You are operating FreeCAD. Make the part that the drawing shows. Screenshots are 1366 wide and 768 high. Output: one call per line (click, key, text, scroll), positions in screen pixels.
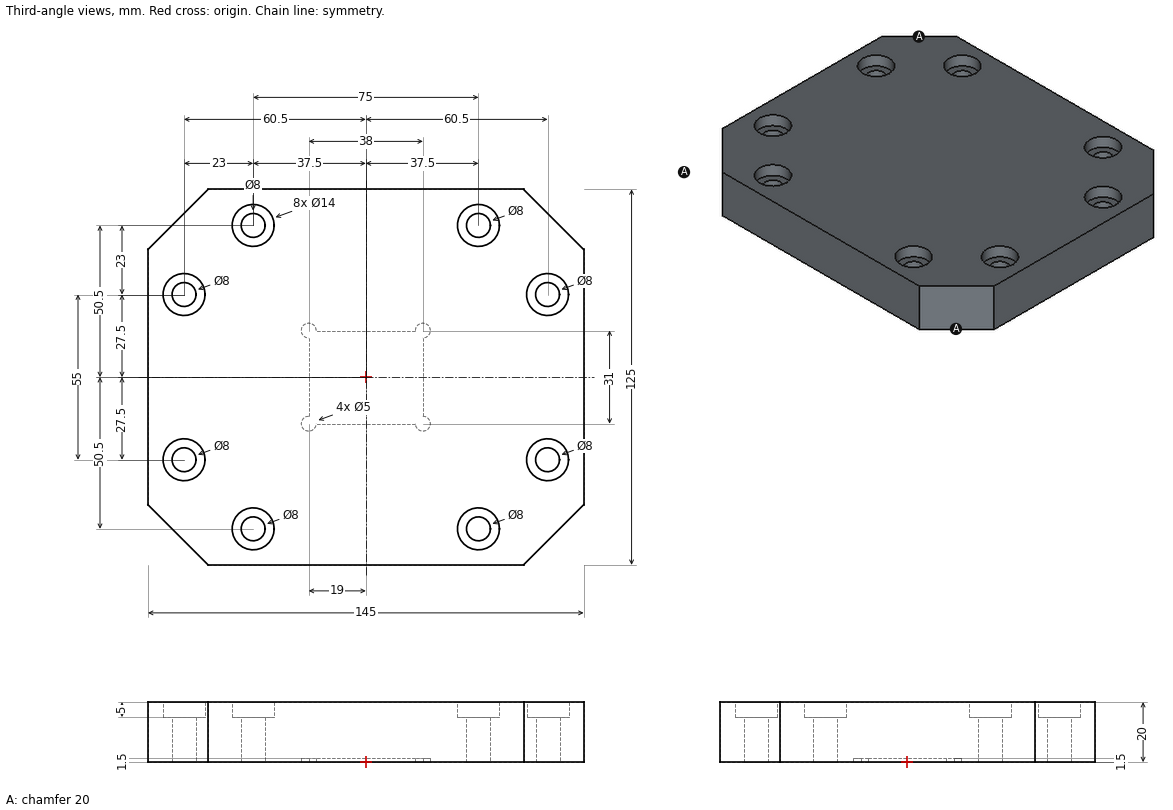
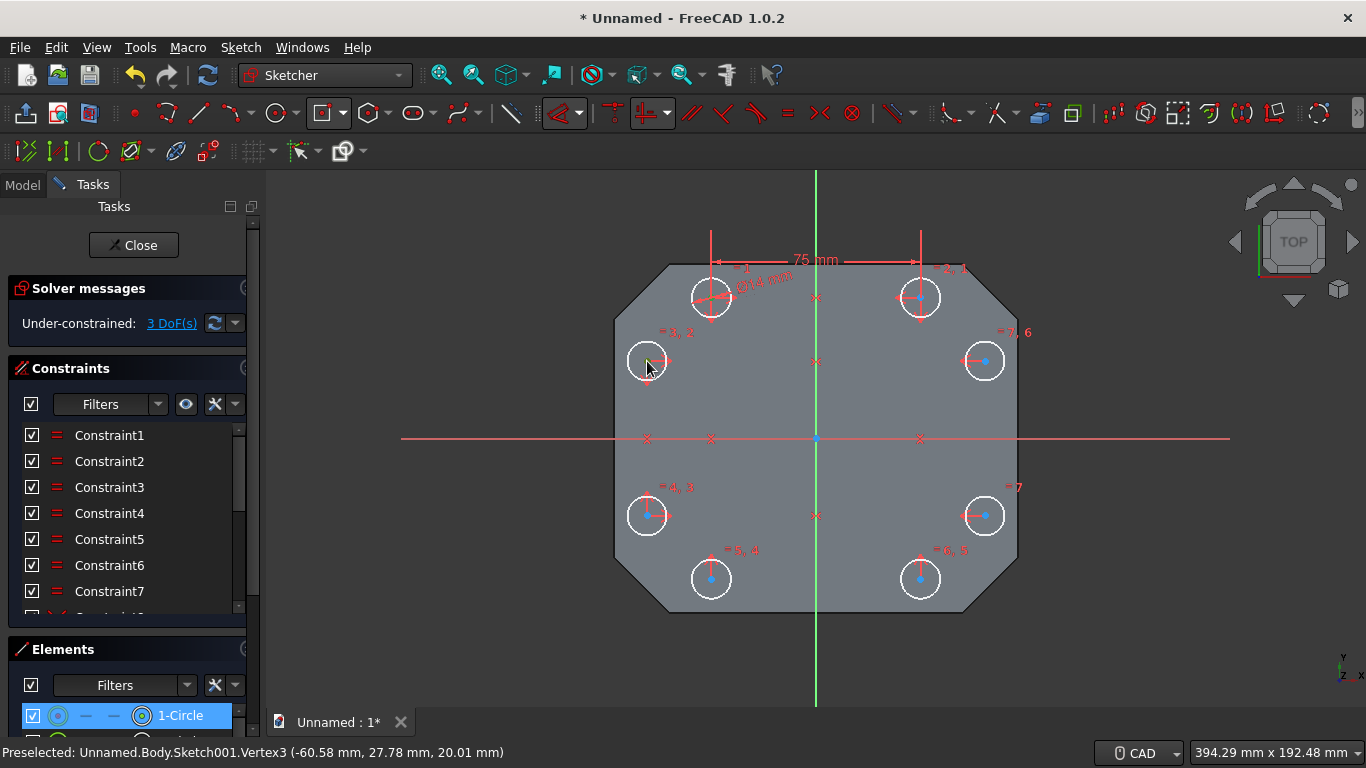
key(l)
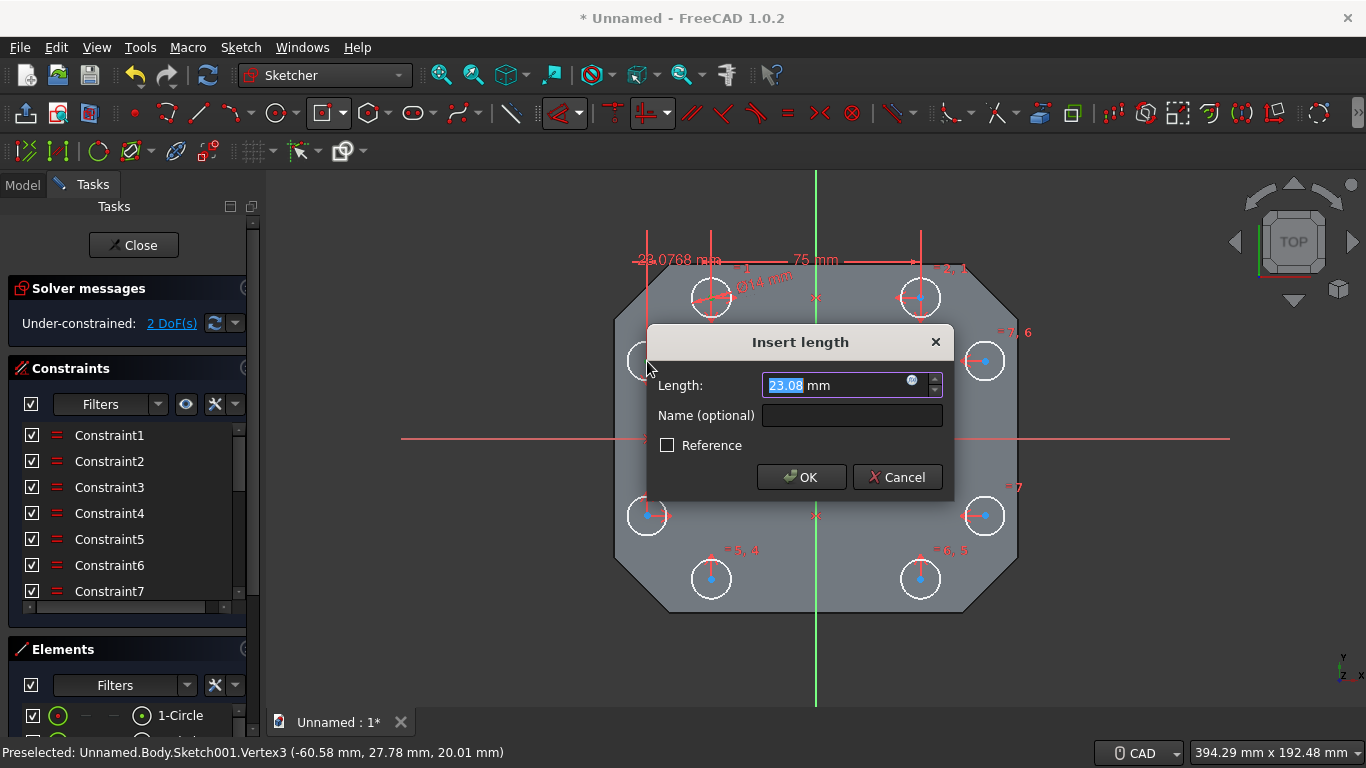
text(23)
key(Return)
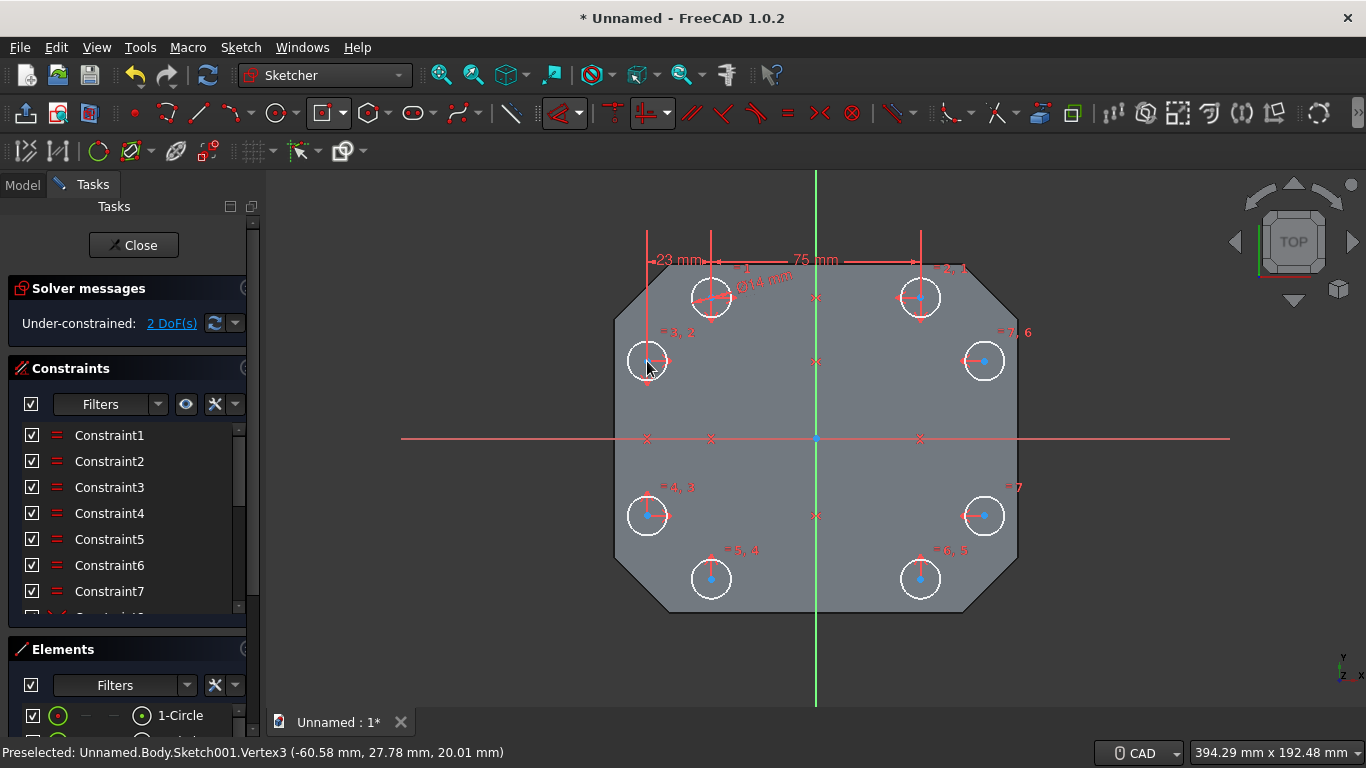
click(711, 298)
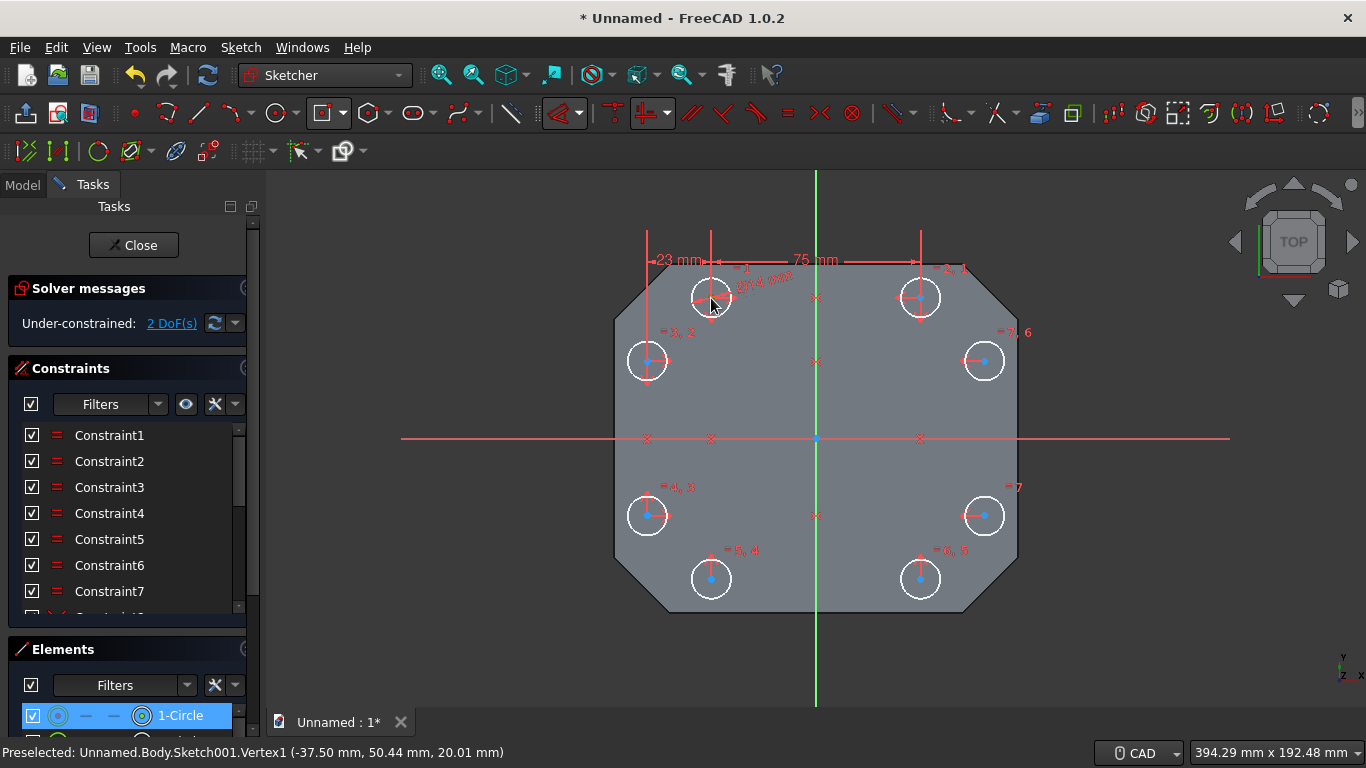
click(647, 361)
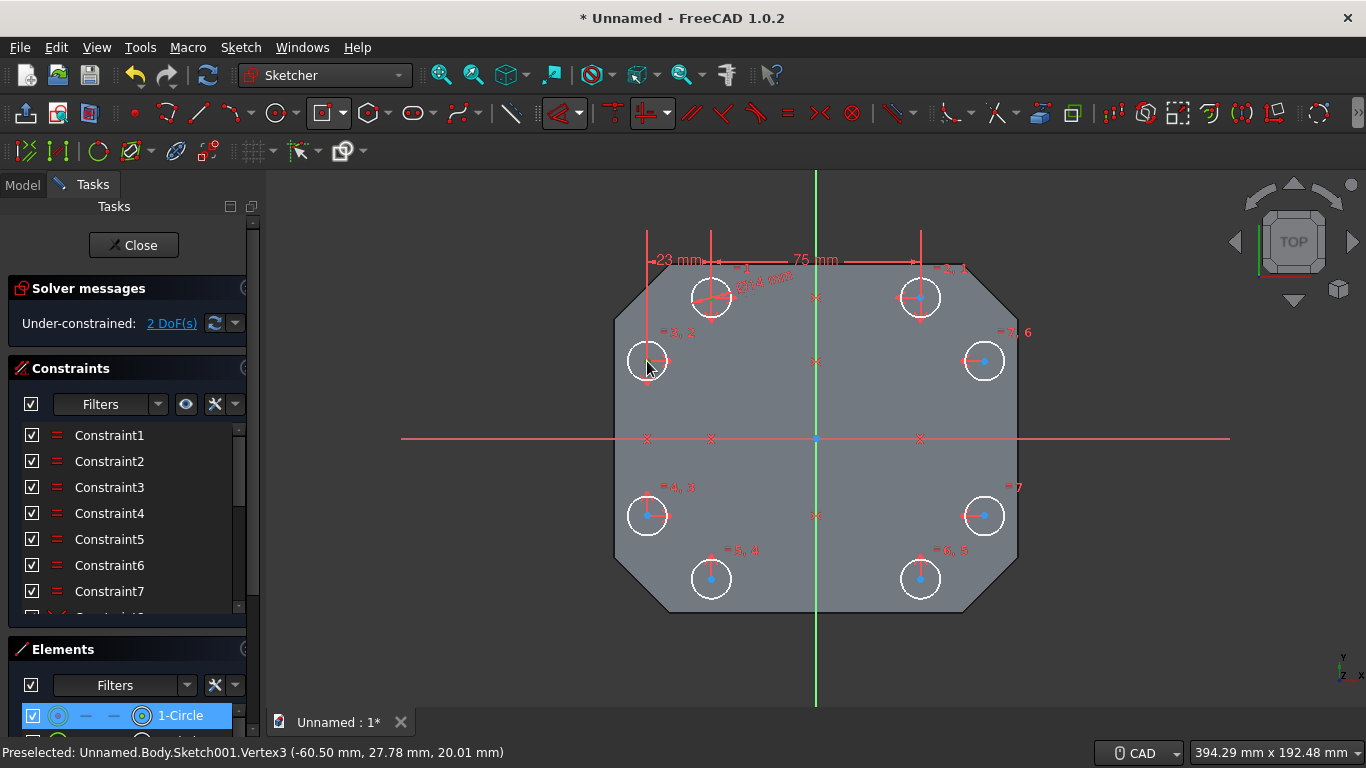
key(i)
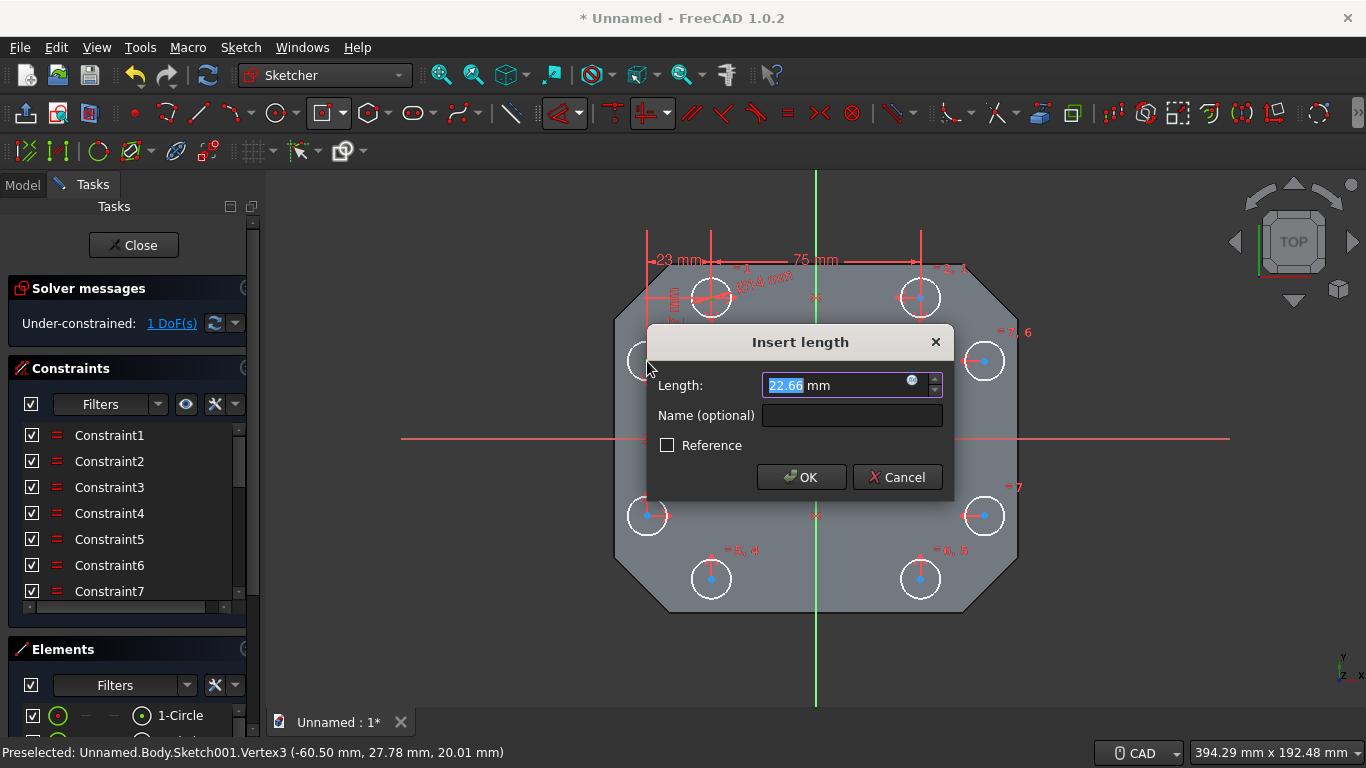
text(23)
key(Return)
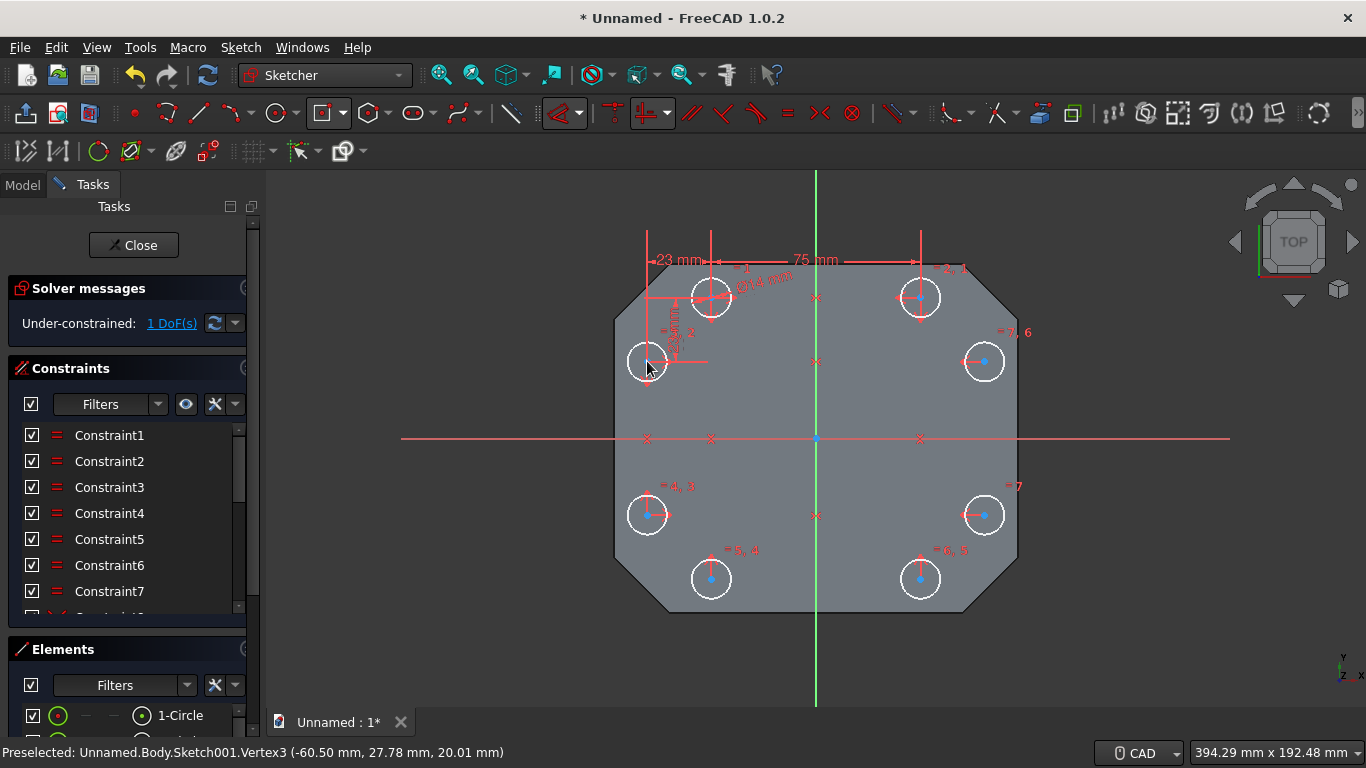
click(647, 362)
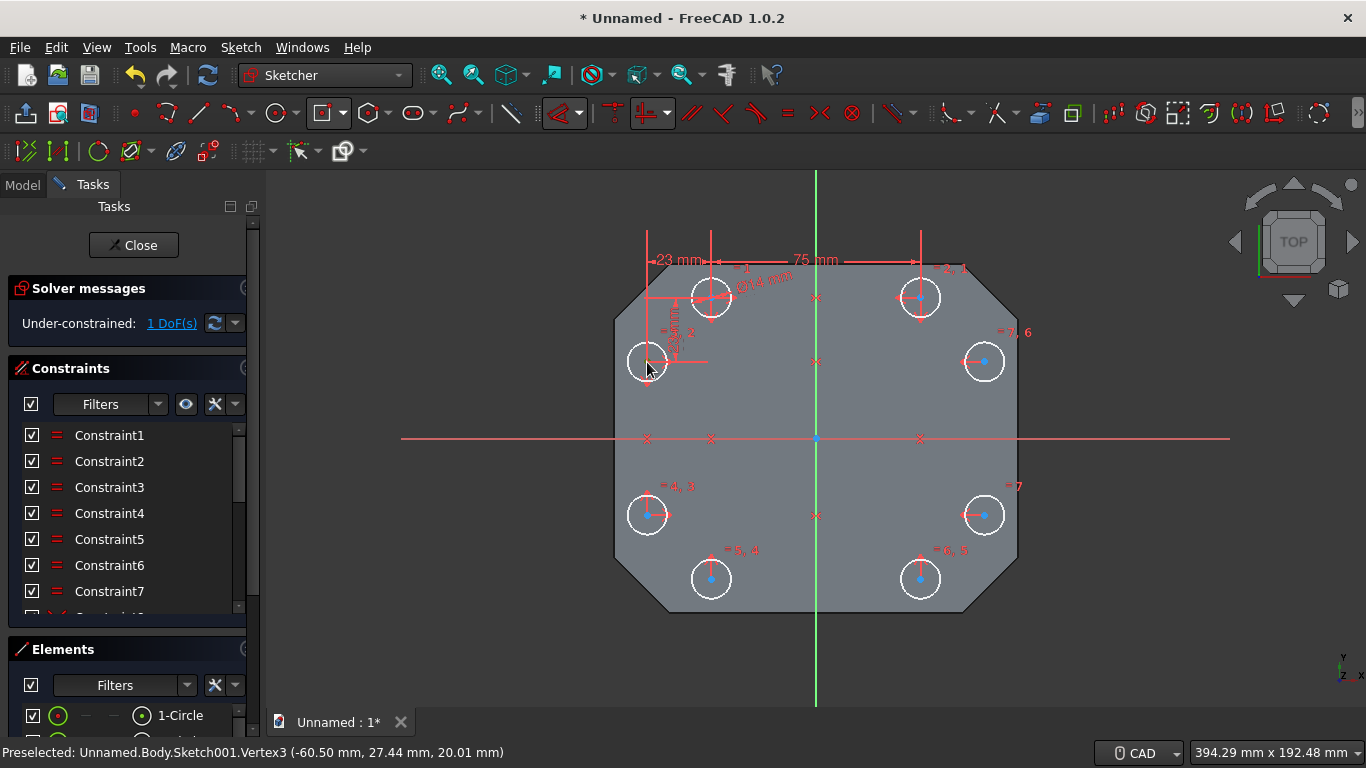
click(647, 515)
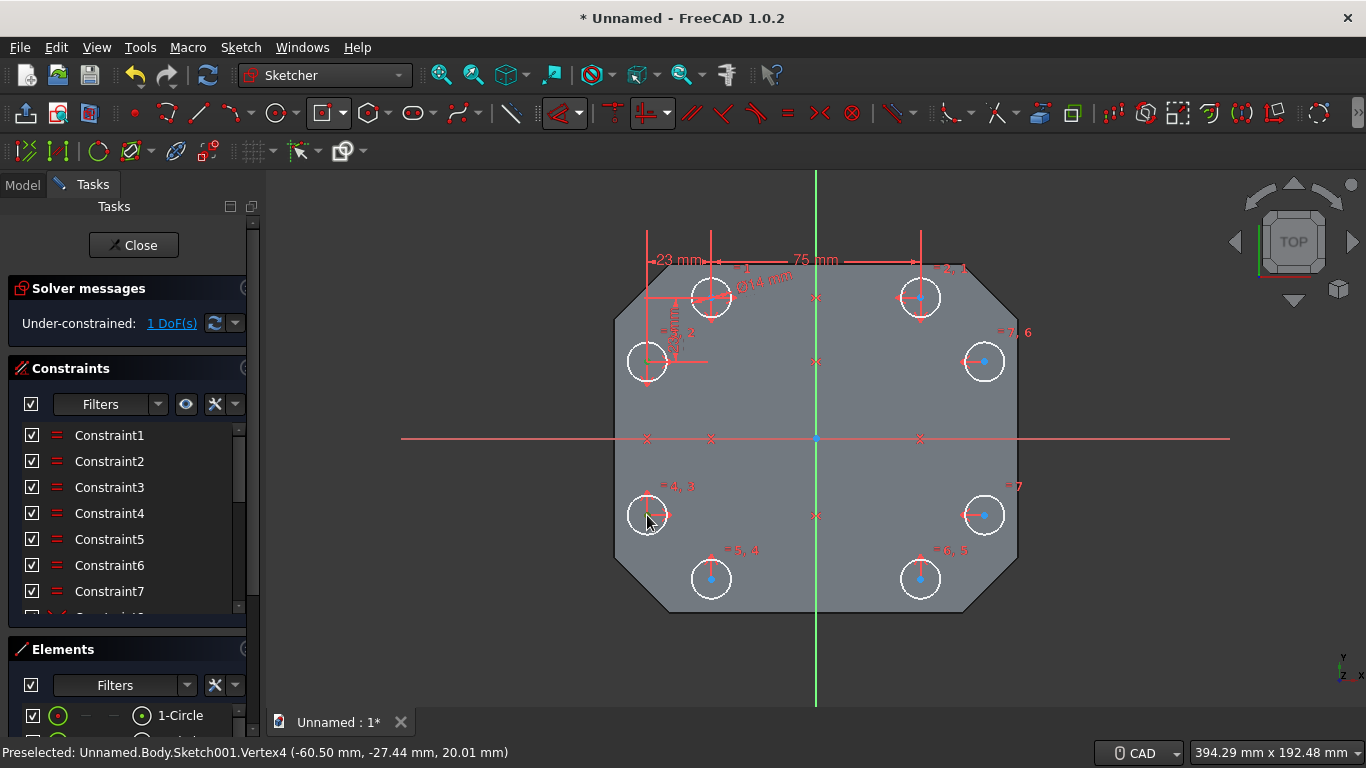
key(i)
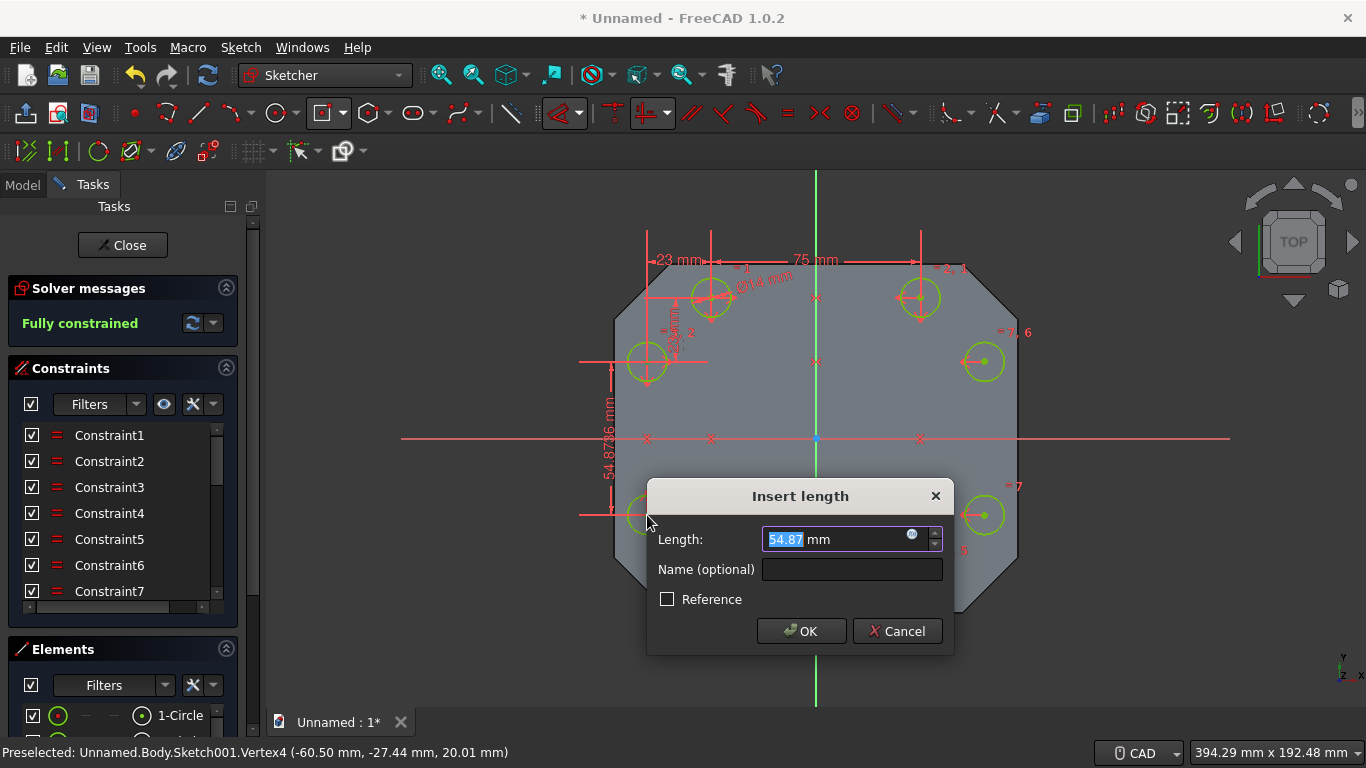
text(55)
key(Return)